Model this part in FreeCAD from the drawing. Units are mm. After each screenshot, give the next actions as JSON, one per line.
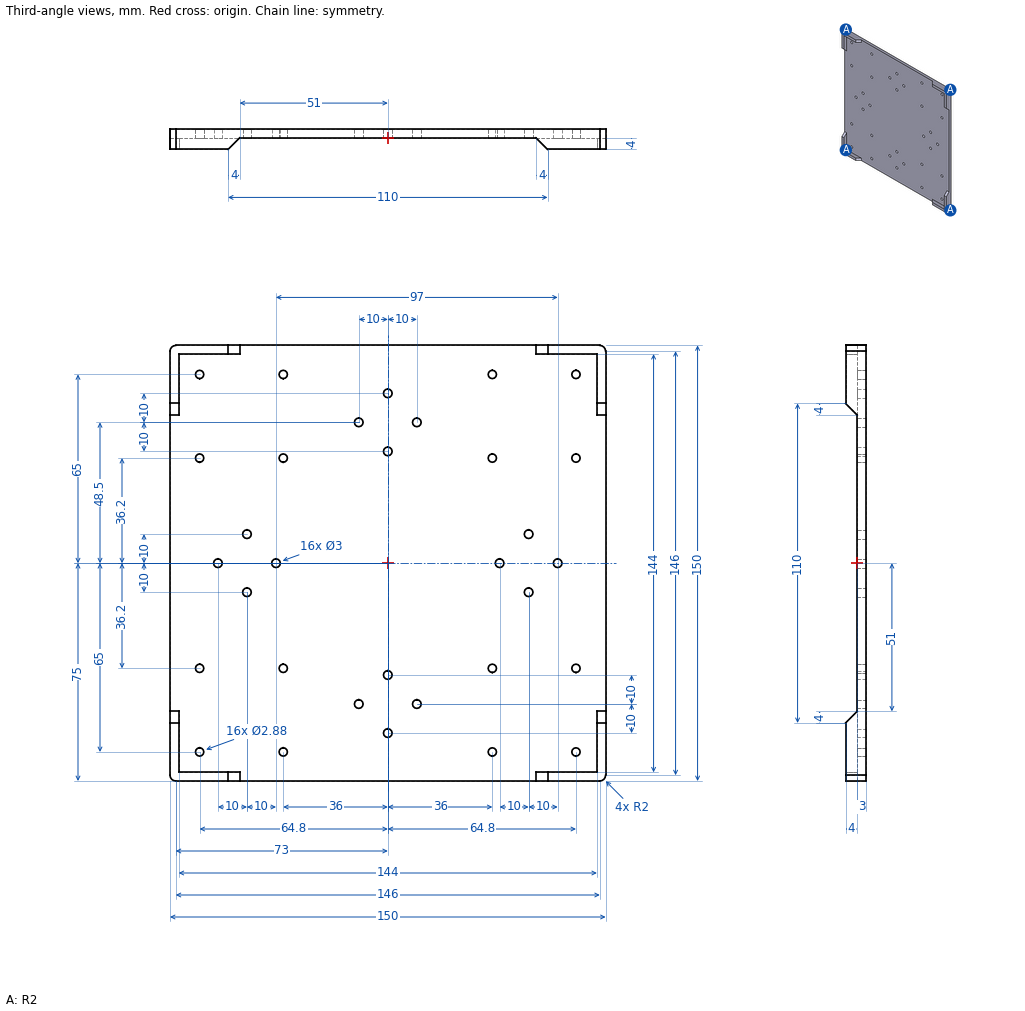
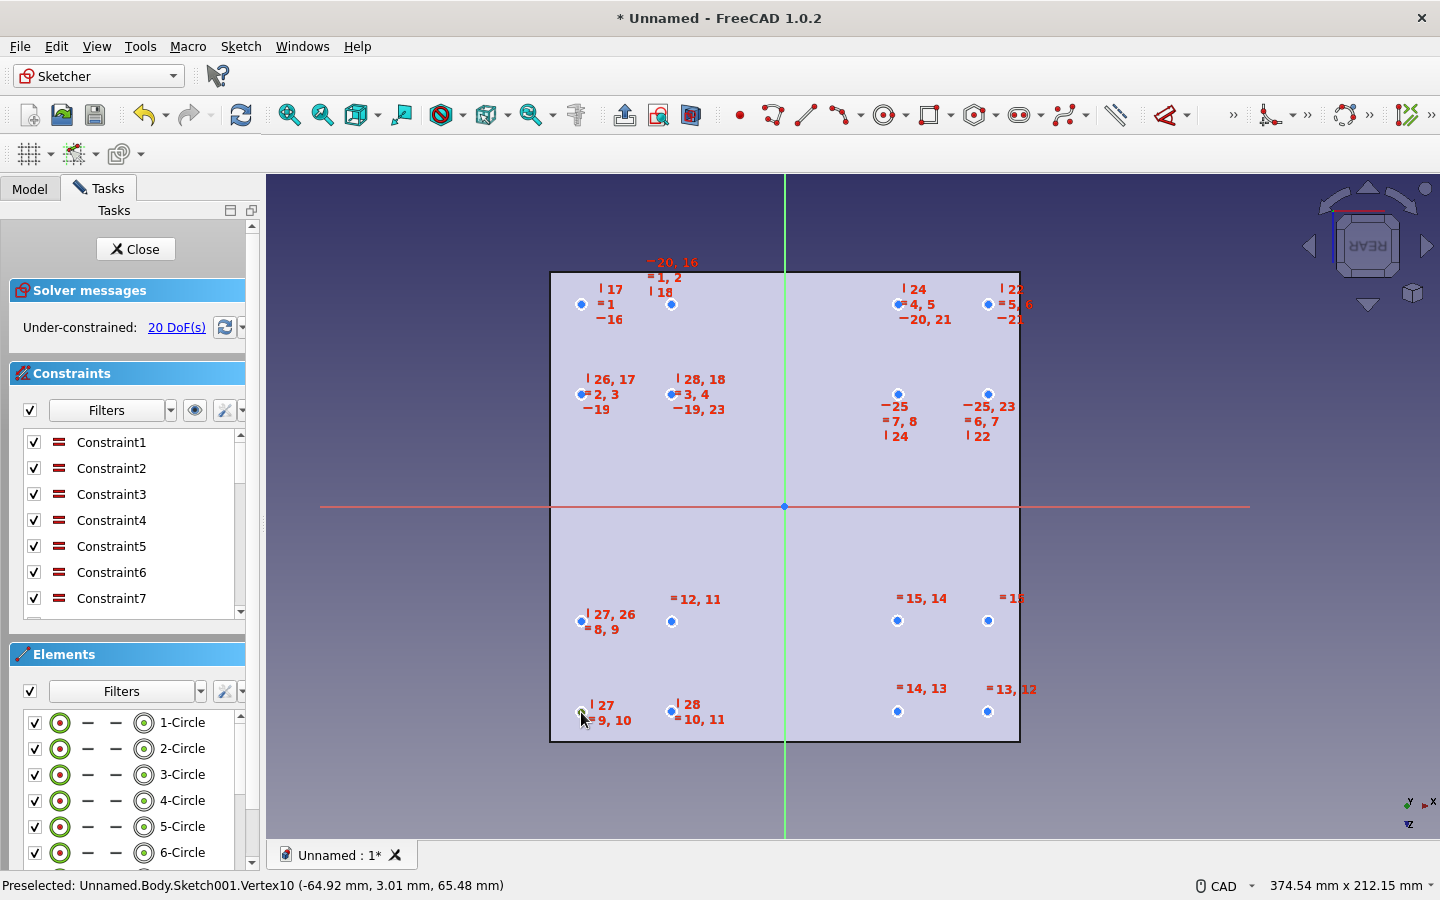
{"action": "left_click", "coordinate": [672, 711]}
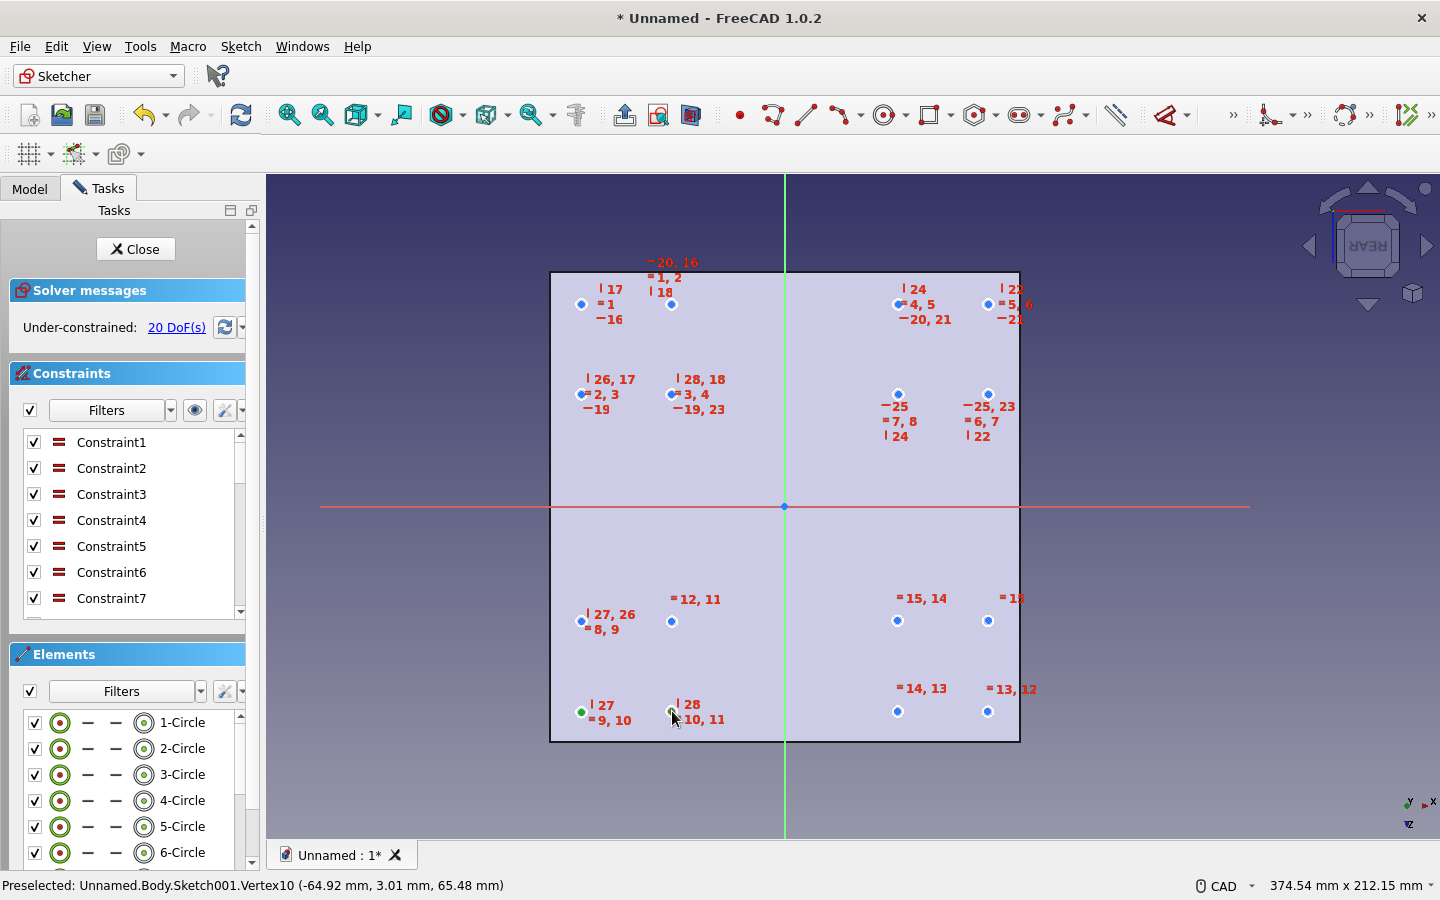
{"action": "key", "text": "h"}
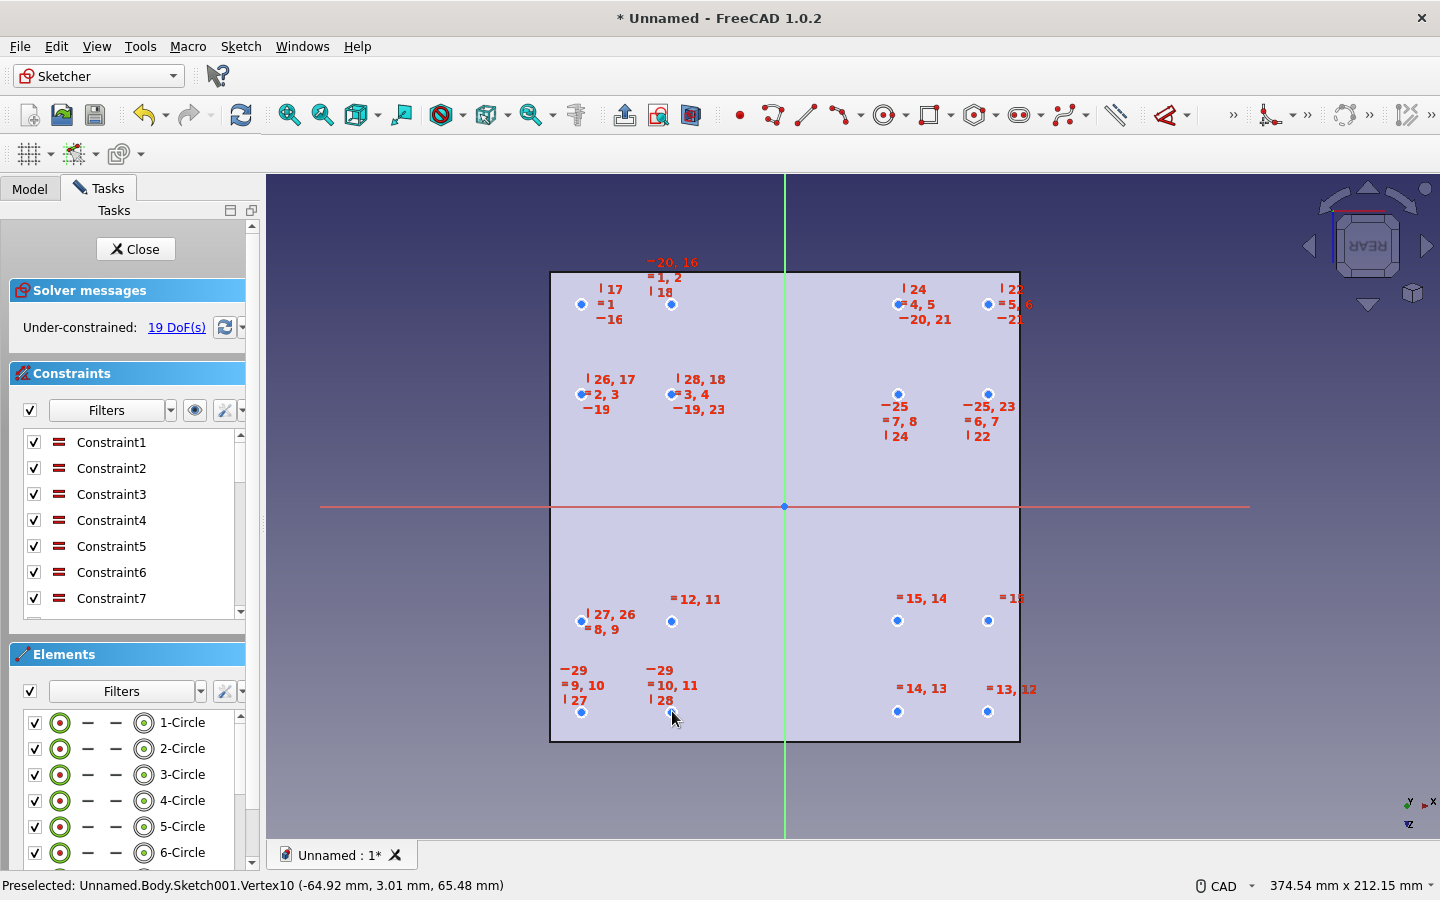
{"action": "left_click", "coordinate": [672, 712]}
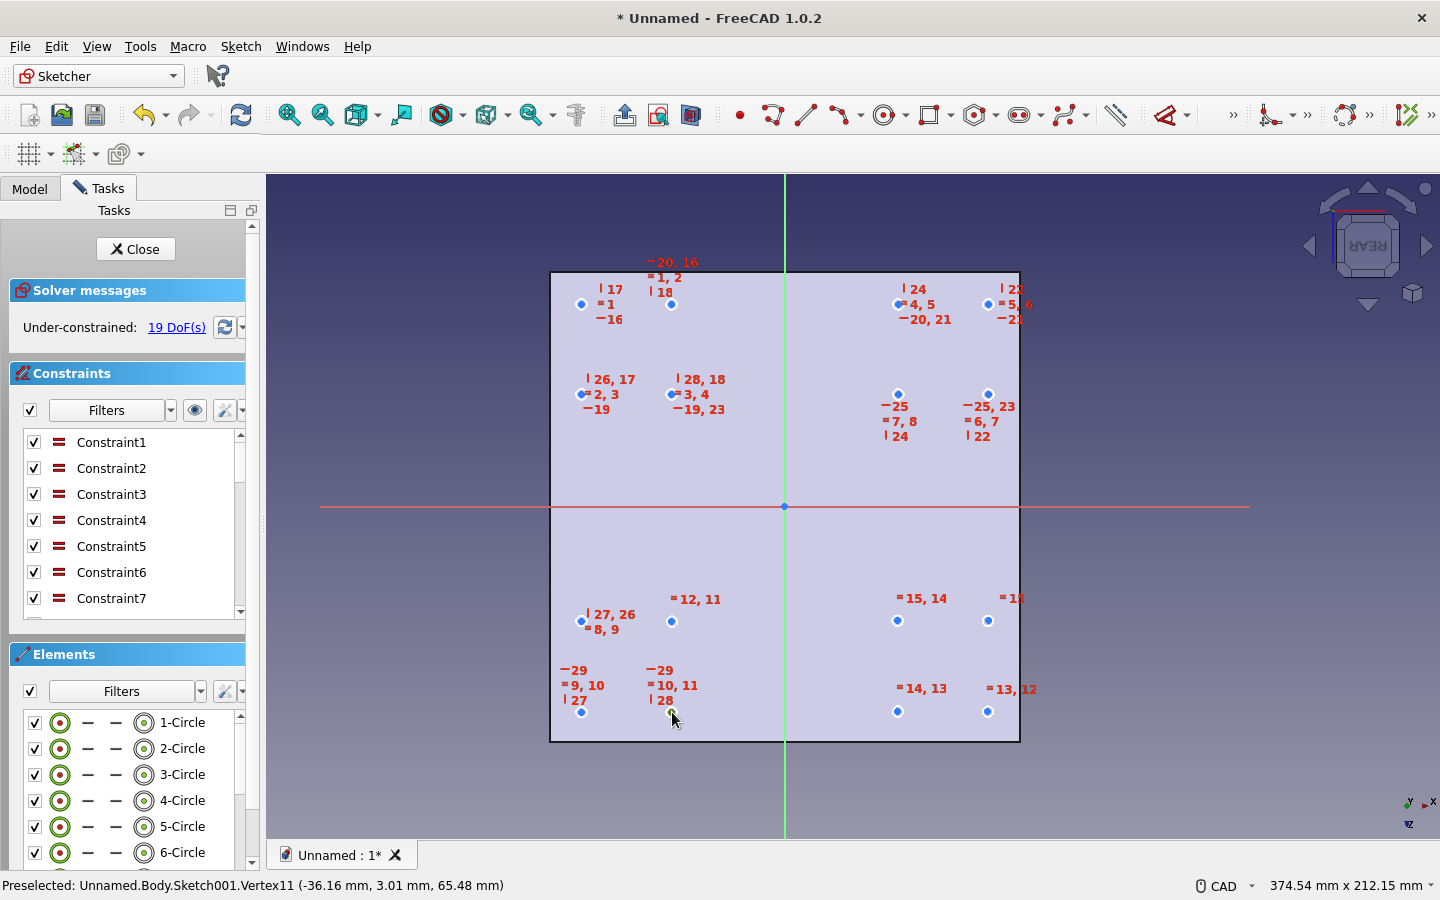
{"action": "left_click", "coordinate": [672, 622]}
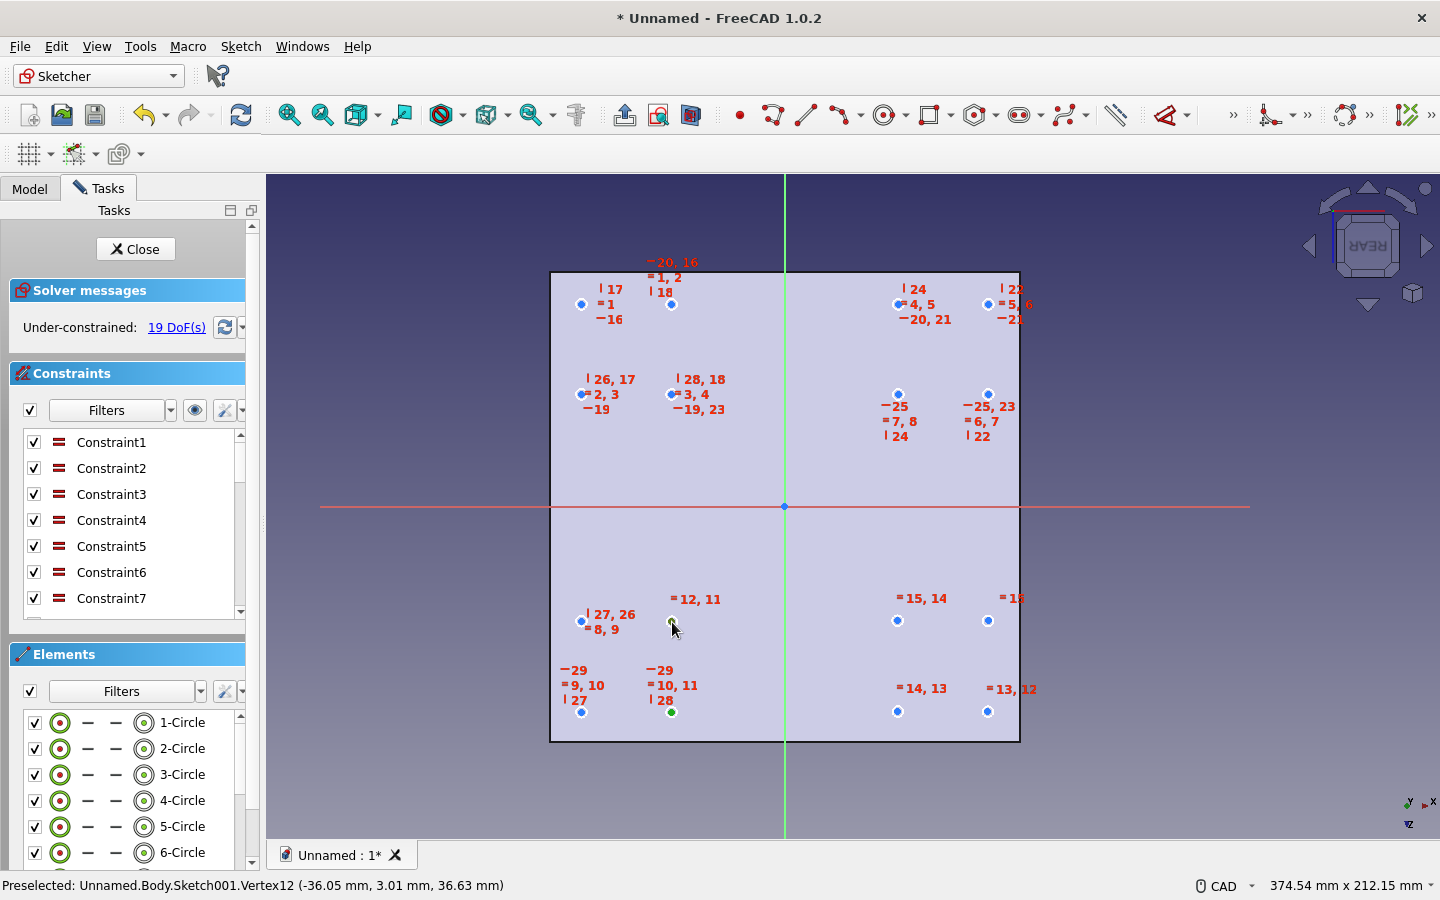
{"action": "key", "text": "v"}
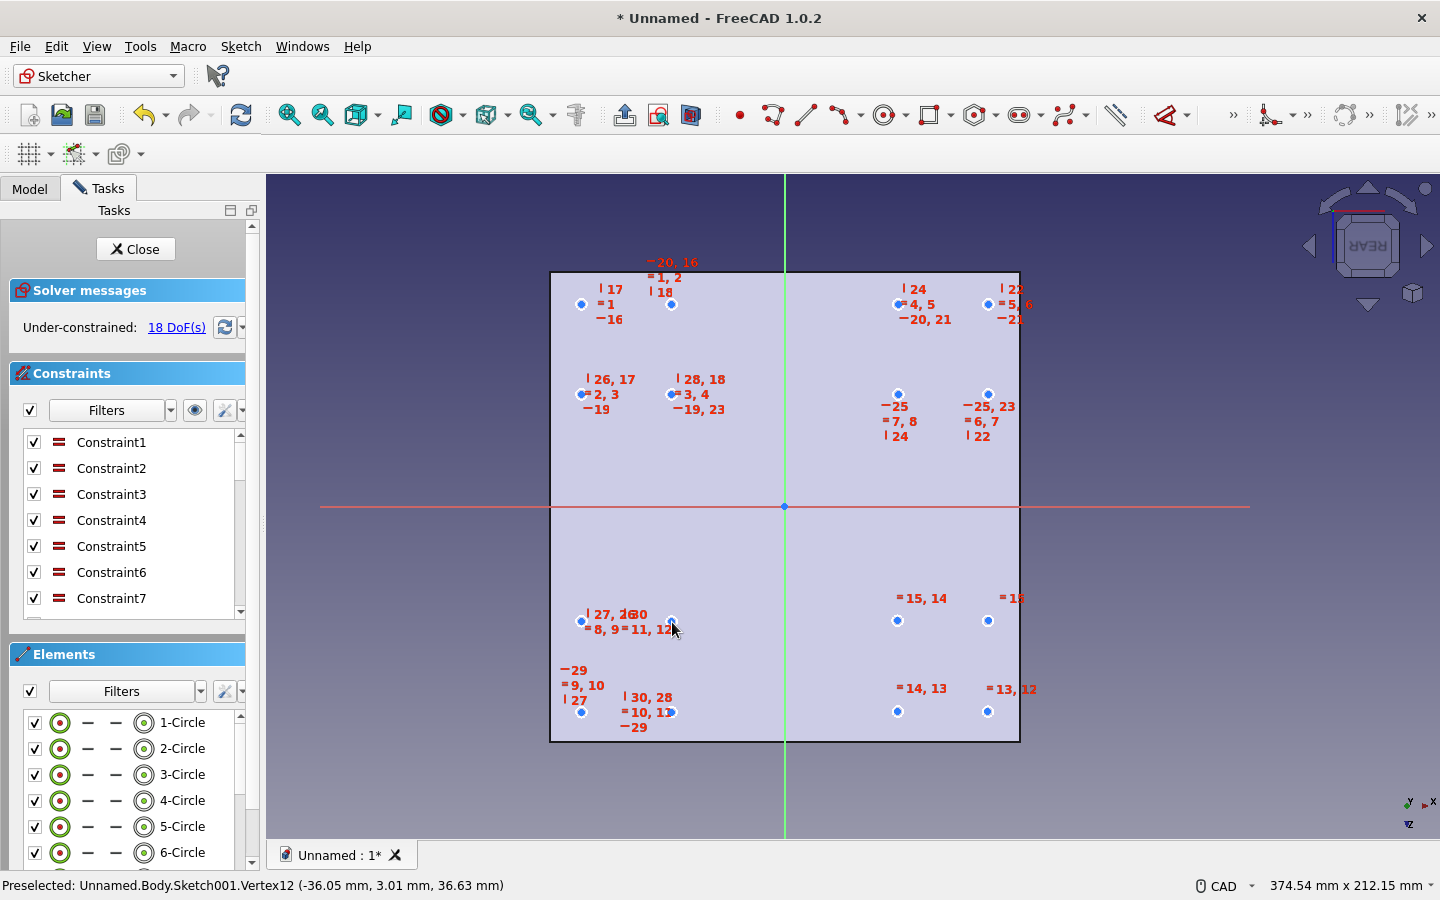
{"action": "left_click", "coordinate": [581, 621]}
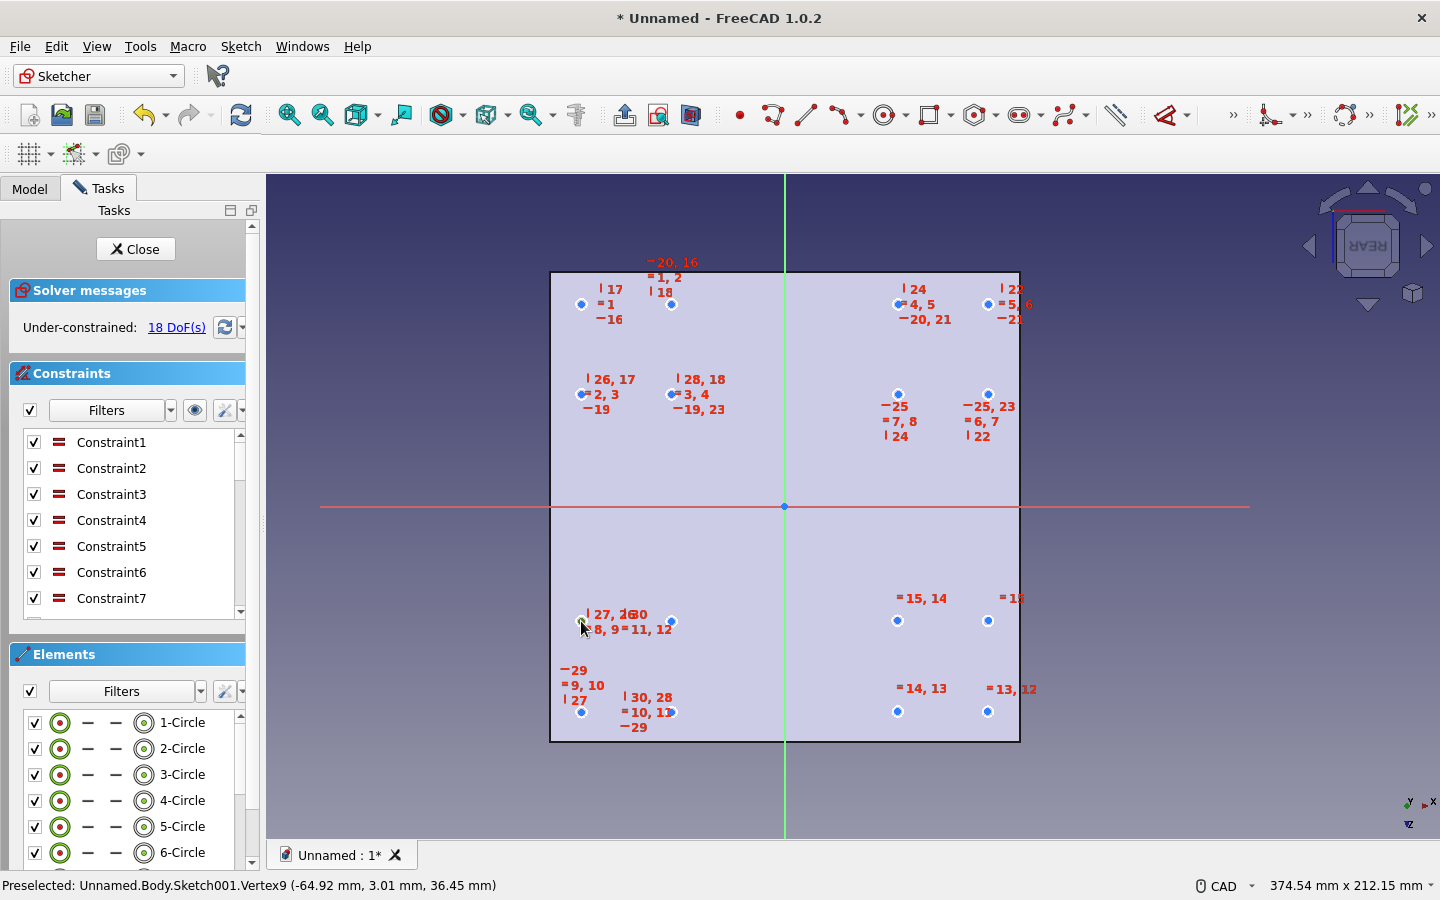
{"action": "left_click", "coordinate": [672, 622]}